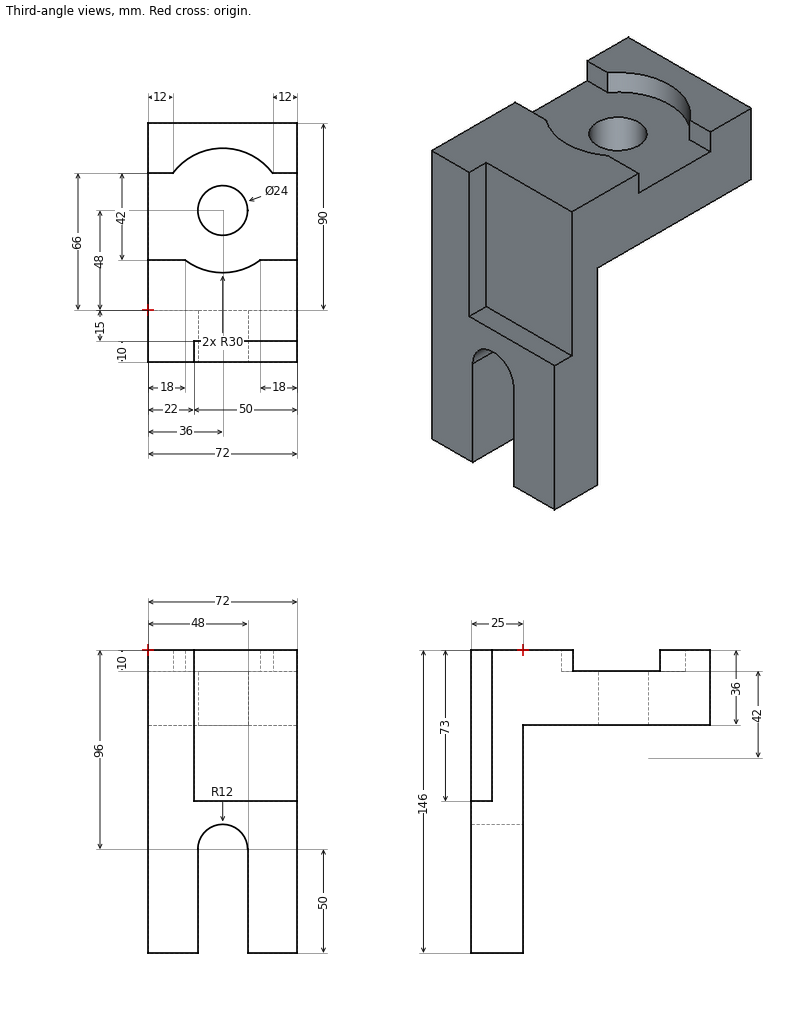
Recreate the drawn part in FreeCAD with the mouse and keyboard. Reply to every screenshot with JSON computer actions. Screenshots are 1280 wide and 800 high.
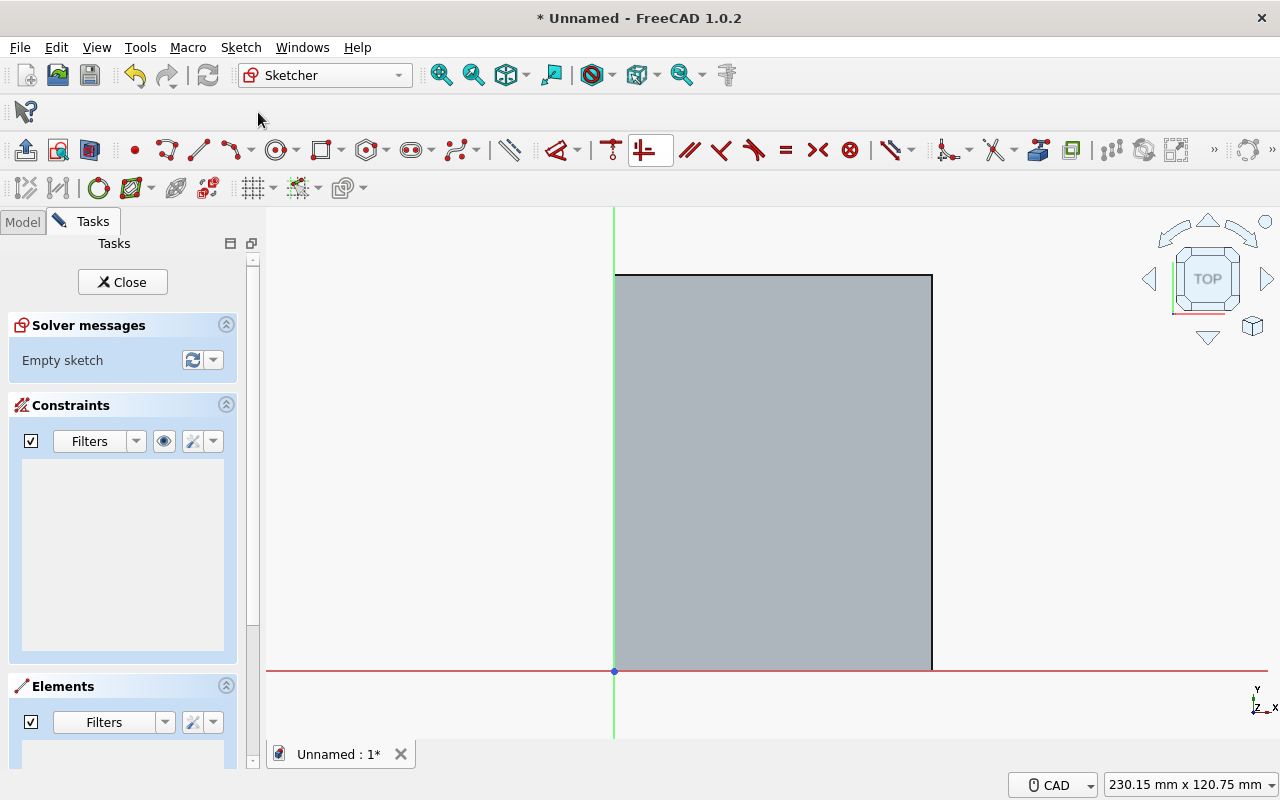
{"action": "left_click", "coordinate": [168, 150]}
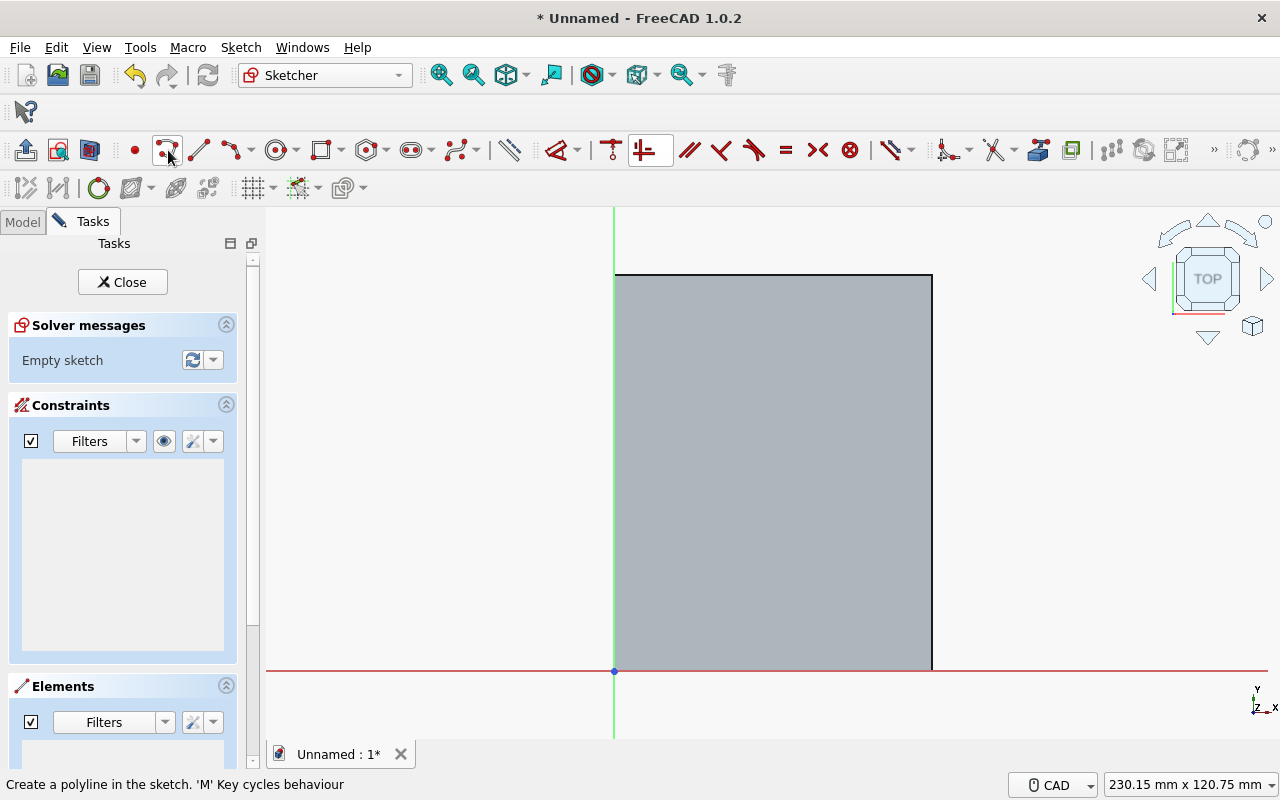
{"action": "left_click", "coordinate": [667, 380]}
{"action": "left_click", "coordinate": [614, 380]}
{"action": "left_click", "coordinate": [623, 566]}
{"action": "left_click", "coordinate": [694, 566]}
{"action": "right_click", "coordinate": [694, 566]}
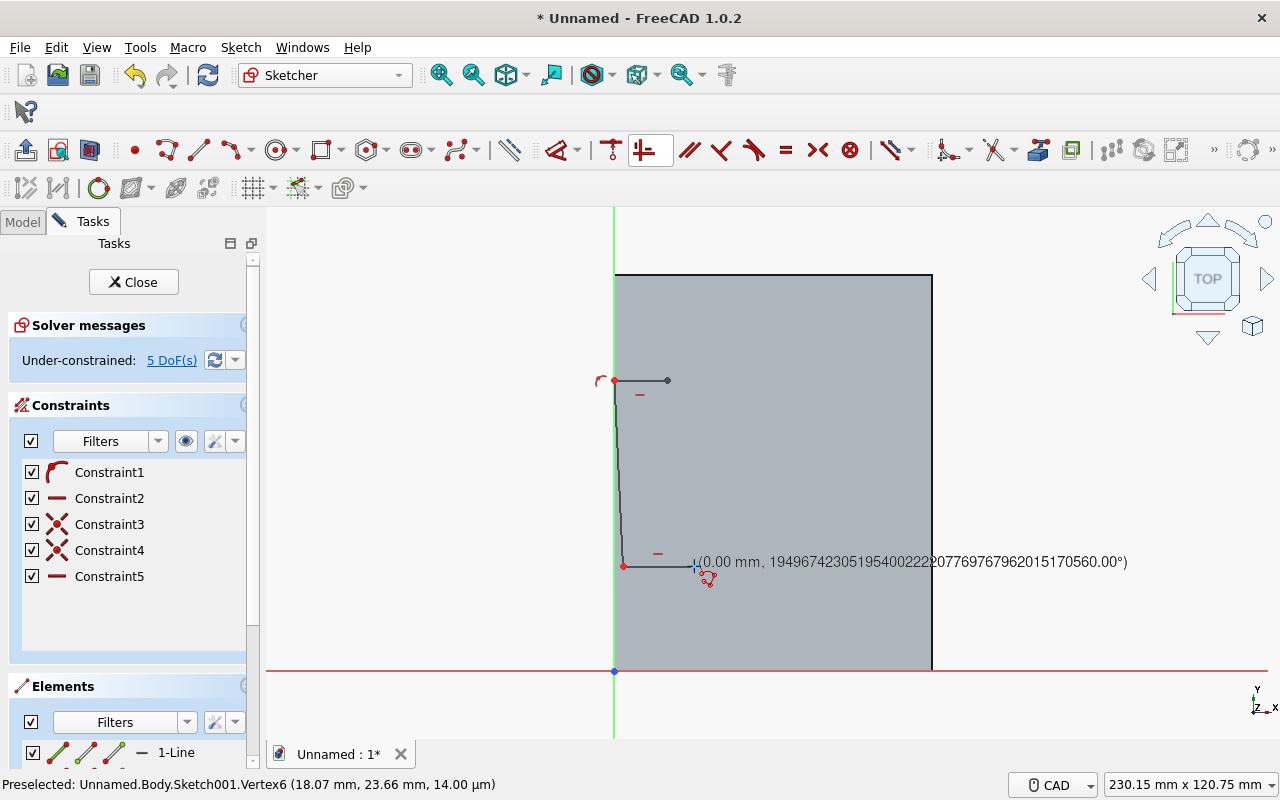
{"action": "left_click", "coordinate": [852, 566]}
{"action": "left_click", "coordinate": [932, 566]}
{"action": "left_click", "coordinate": [932, 380]}
{"action": "left_click", "coordinate": [879, 380]}
{"action": "right_click", "coordinate": [879, 380]}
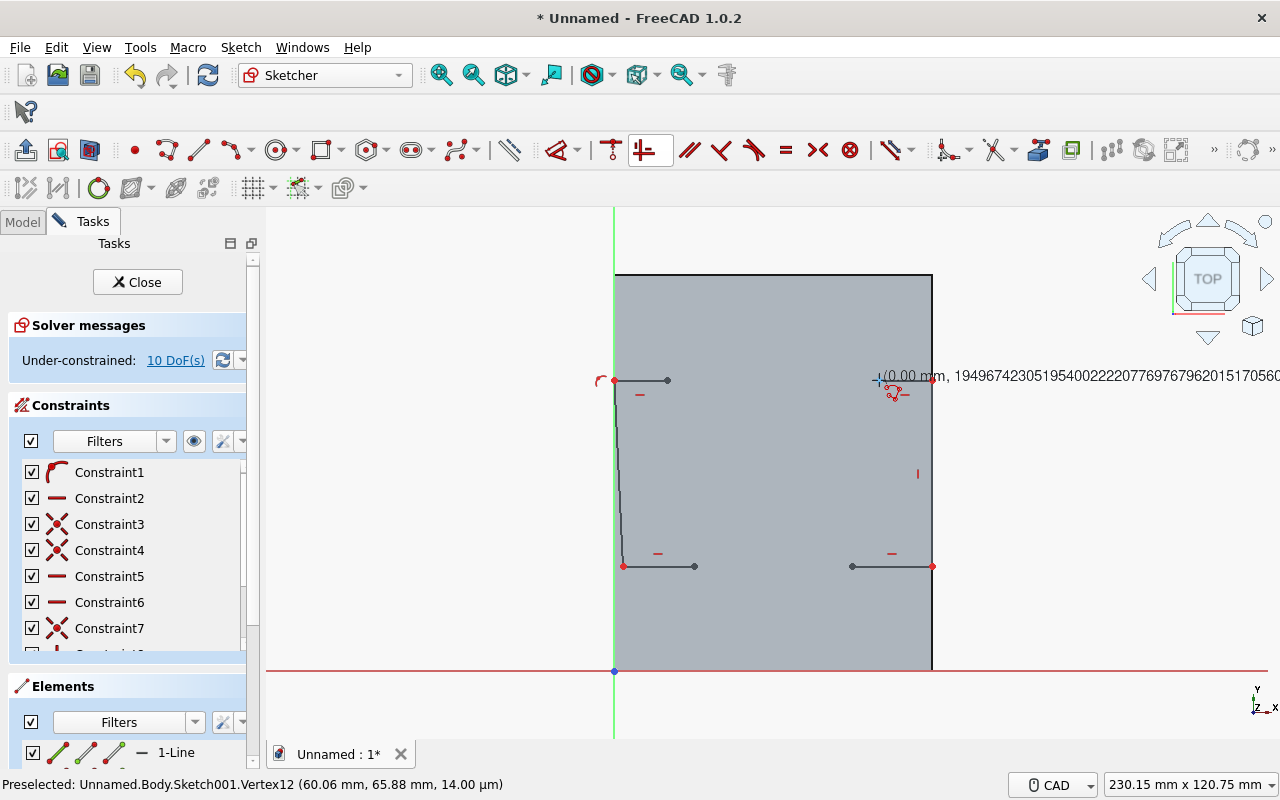
{"action": "left_click", "coordinate": [232, 150]}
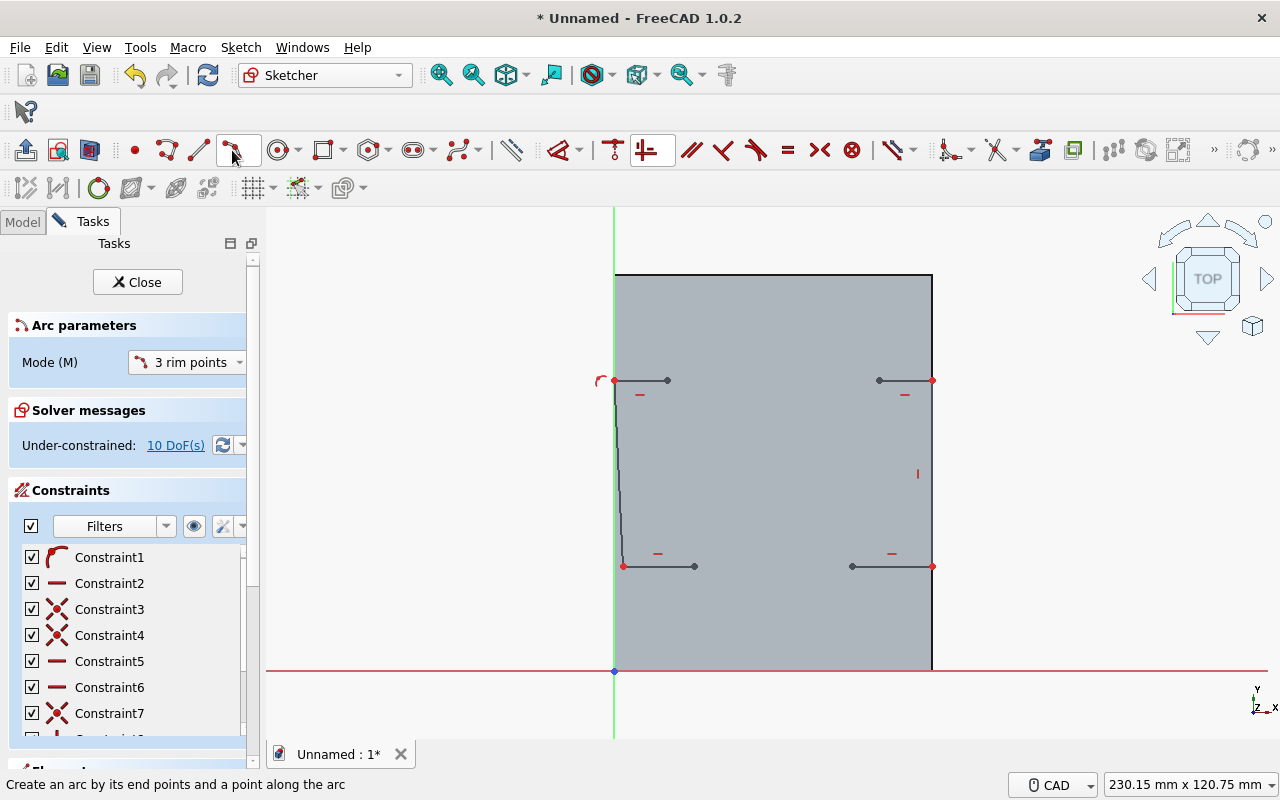
{"action": "left_click", "coordinate": [694, 567]}
{"action": "left_click", "coordinate": [852, 567]}
{"action": "left_click", "coordinate": [773, 592]}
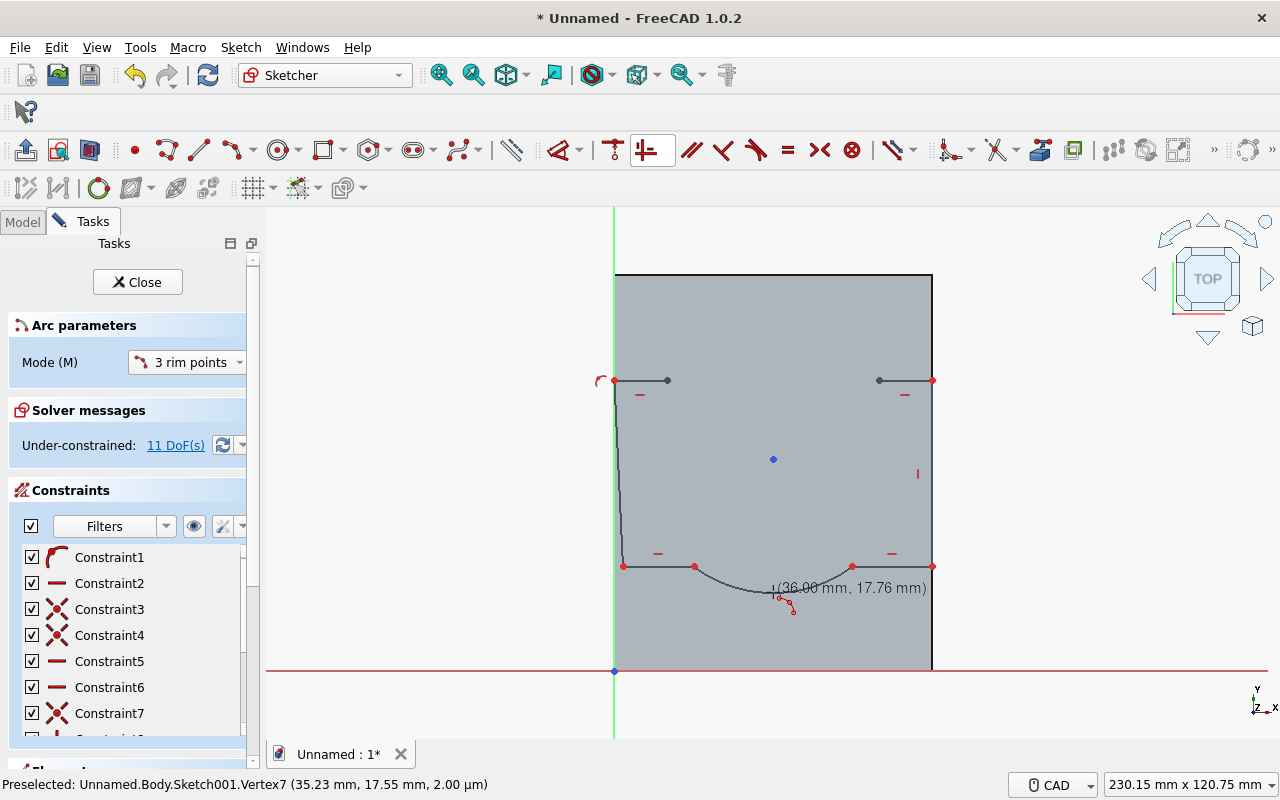
{"action": "left_click", "coordinate": [879, 381]}
{"action": "left_click", "coordinate": [667, 381]}
{"action": "left_click", "coordinate": [773, 328]}
{"action": "key", "text": "Escape"}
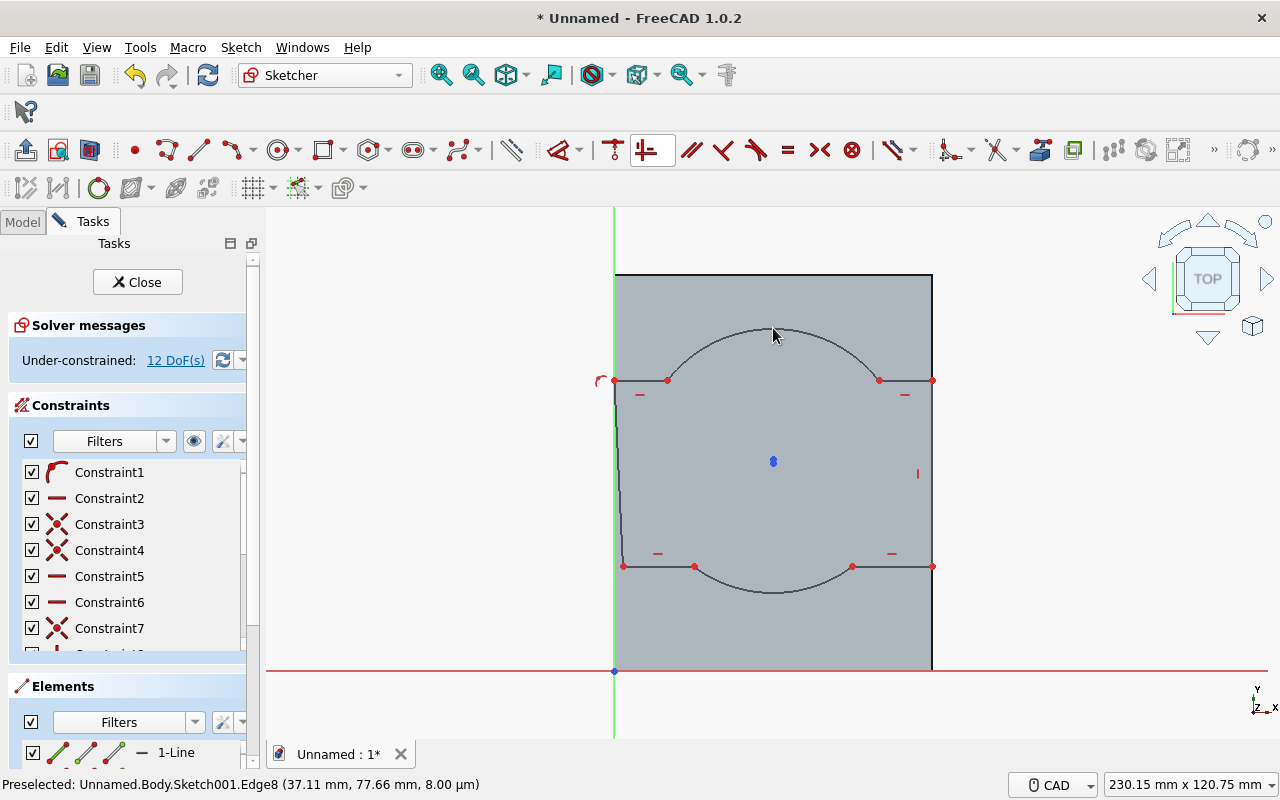
{"action": "left_click", "coordinate": [617, 437]}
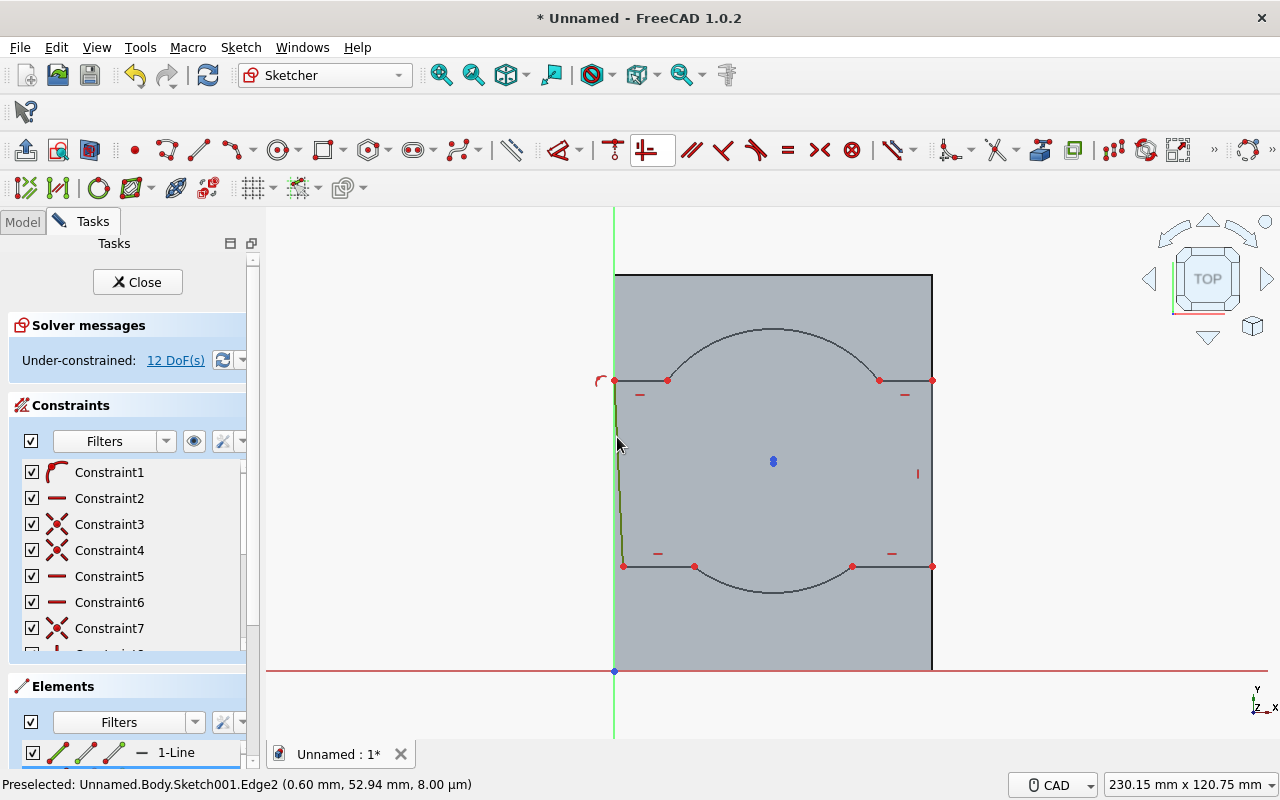
{"action": "key", "text": "v"}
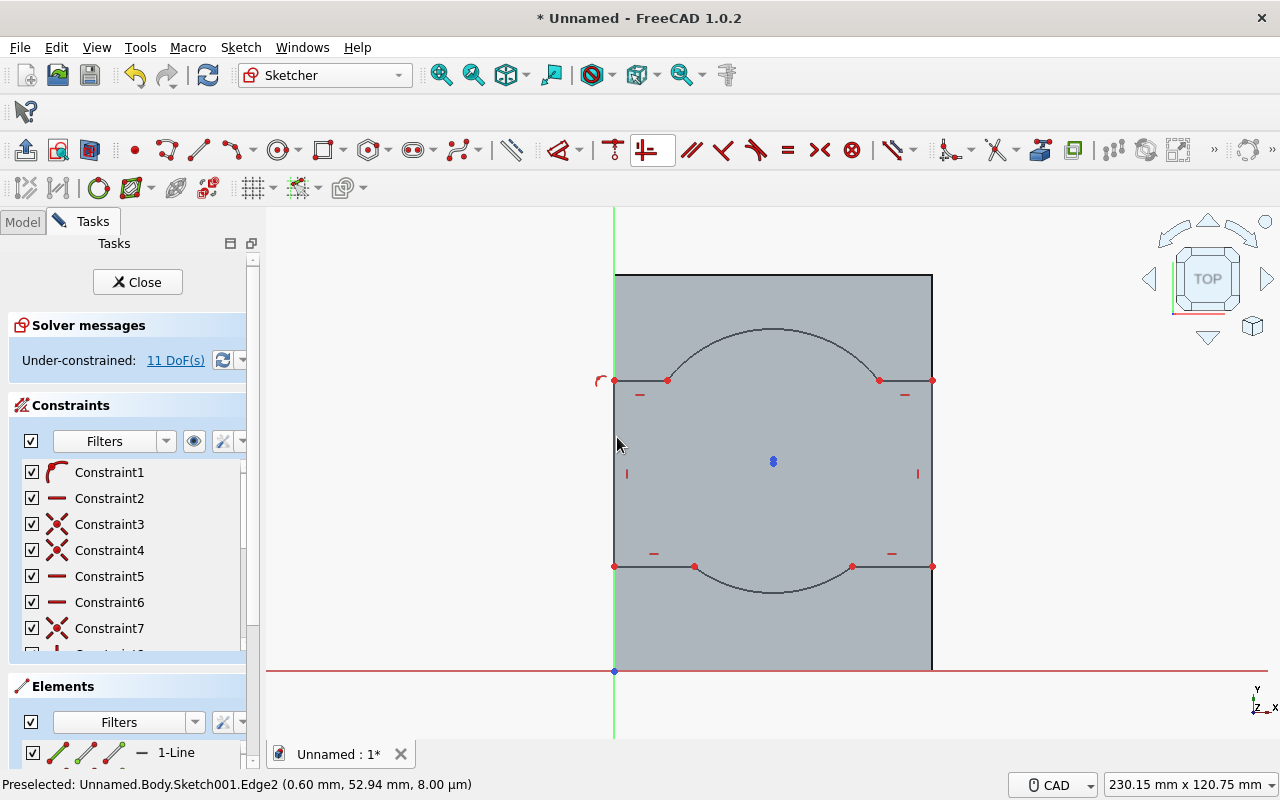
{"action": "left_click", "coordinate": [740, 589]}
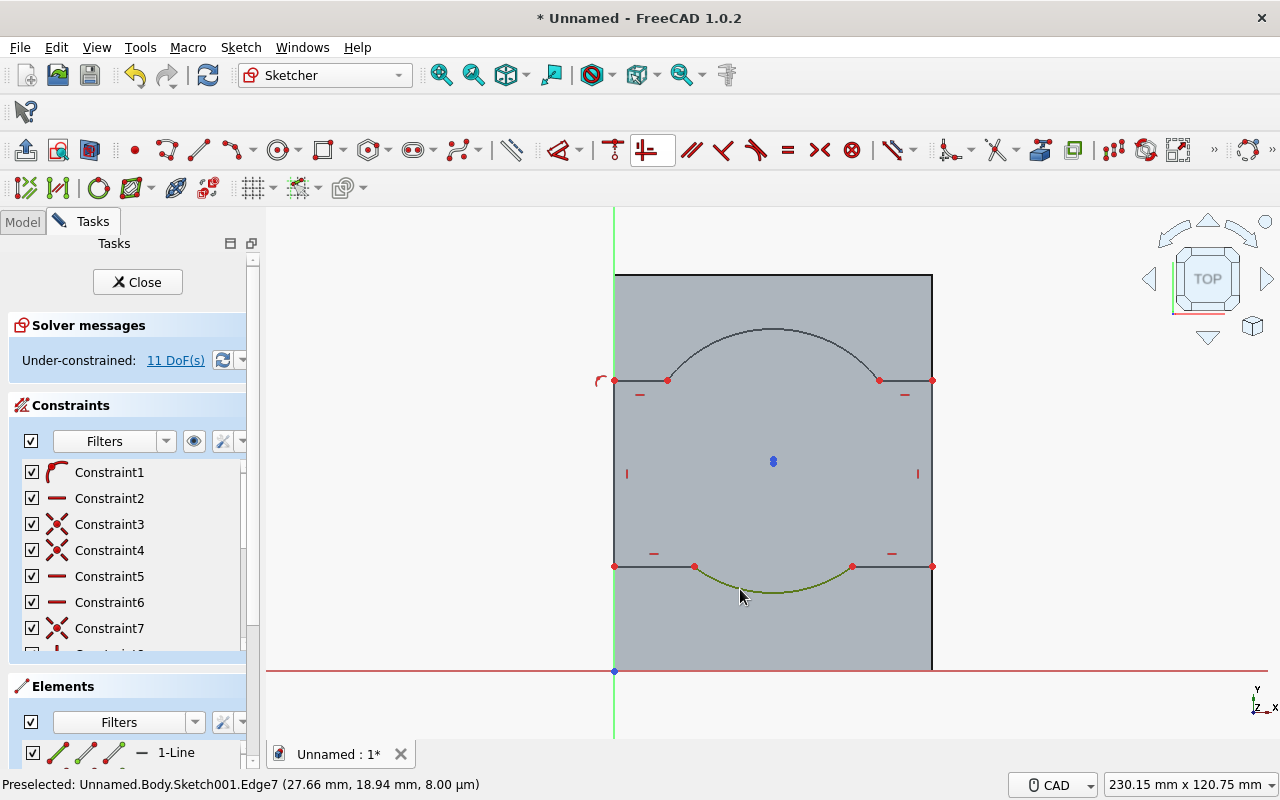
{"action": "left_click", "coordinate": [821, 338]}